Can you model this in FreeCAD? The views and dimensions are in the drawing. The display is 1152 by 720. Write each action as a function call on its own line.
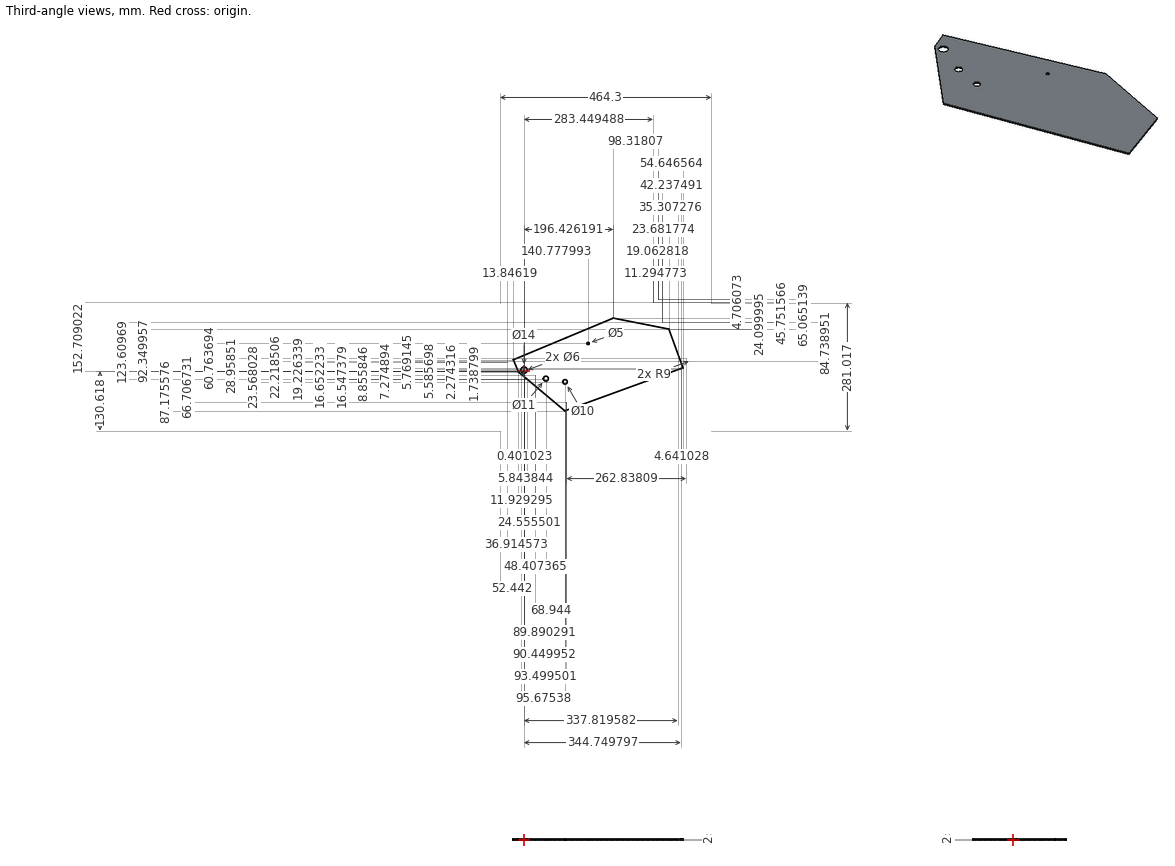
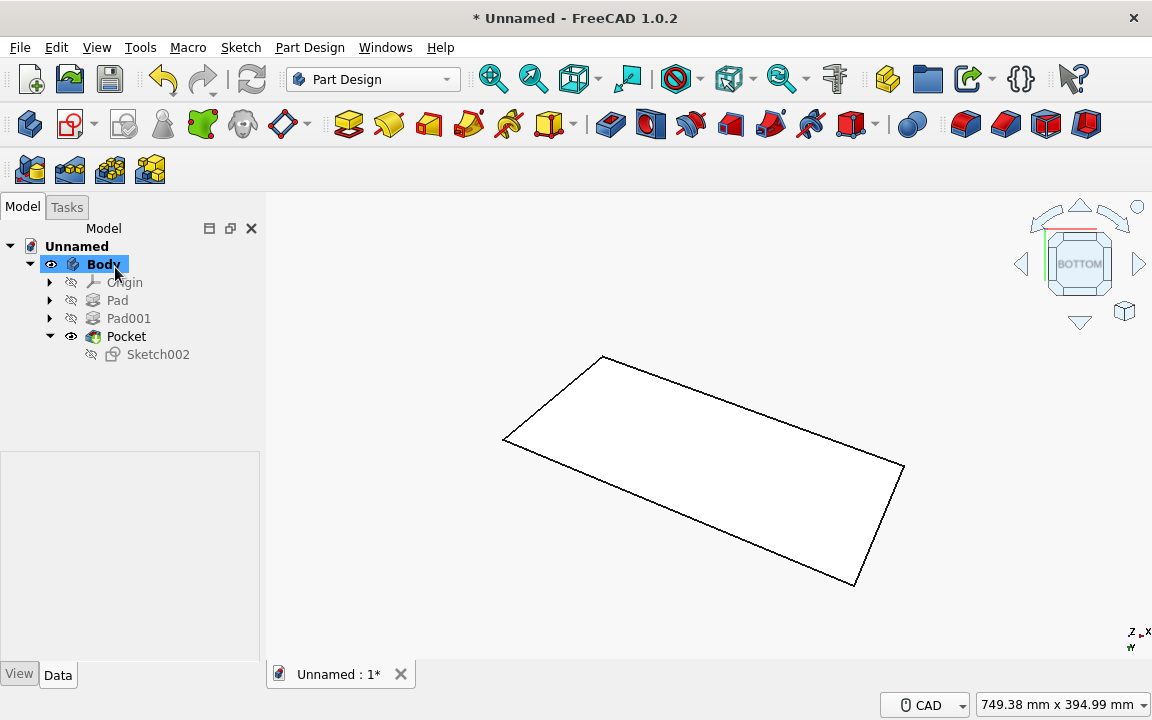
click(70, 124)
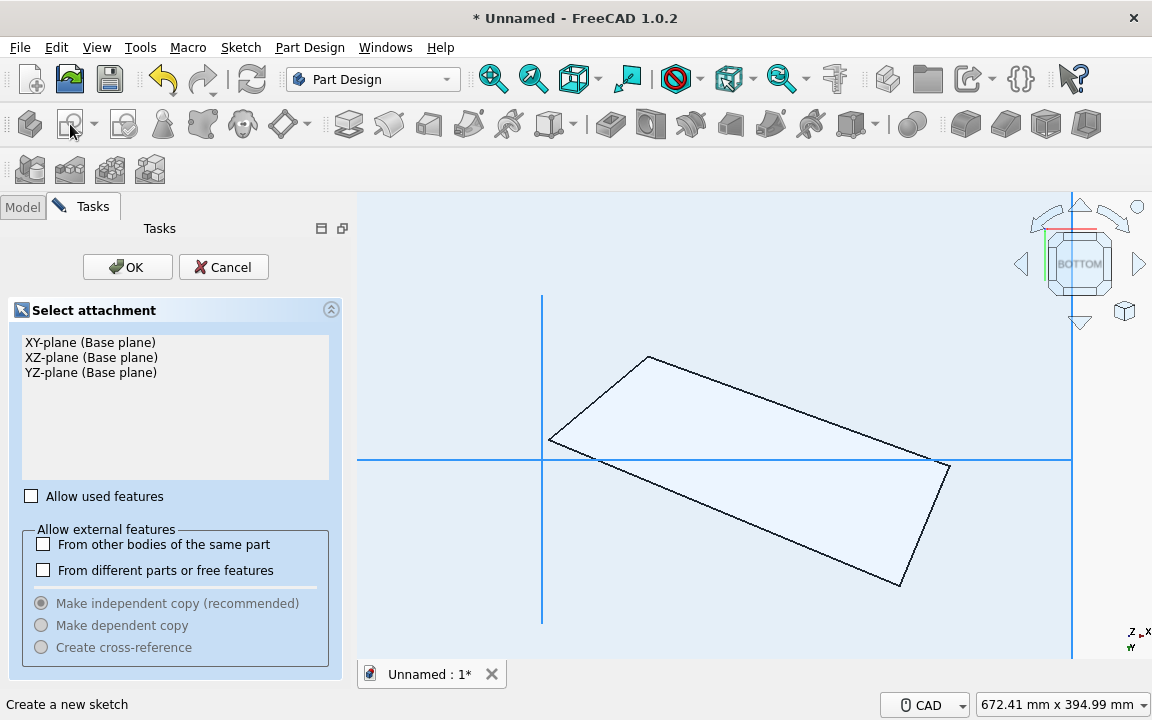
click(82, 342)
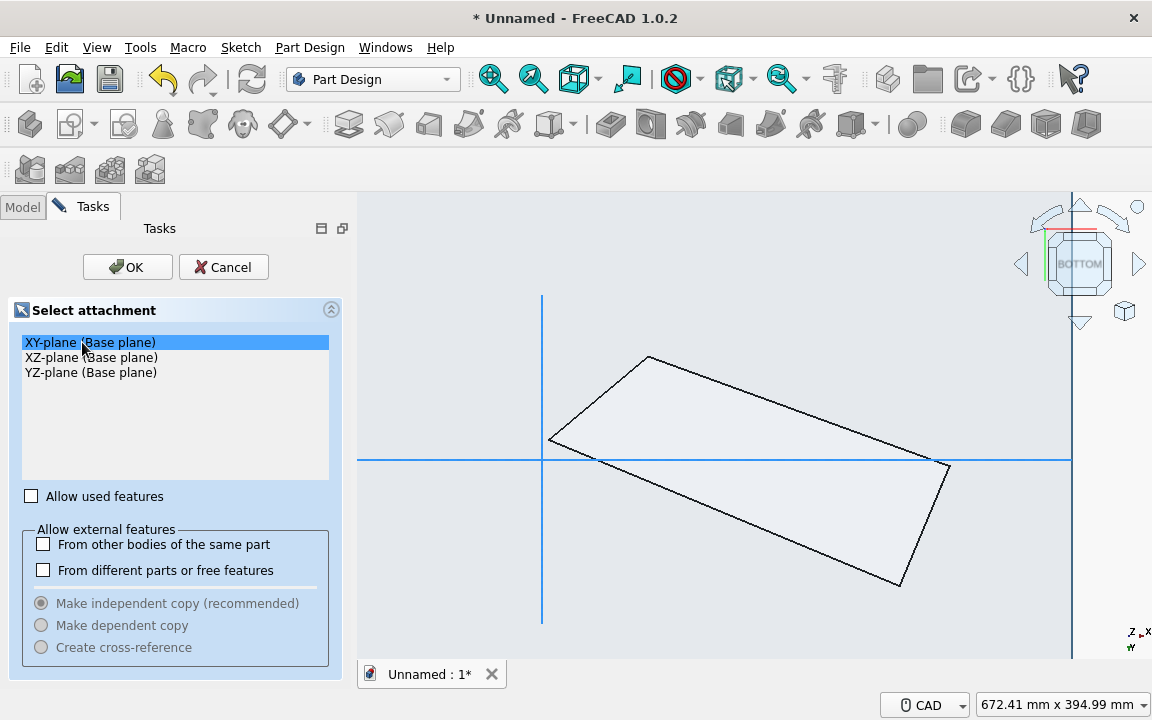
click(128, 267)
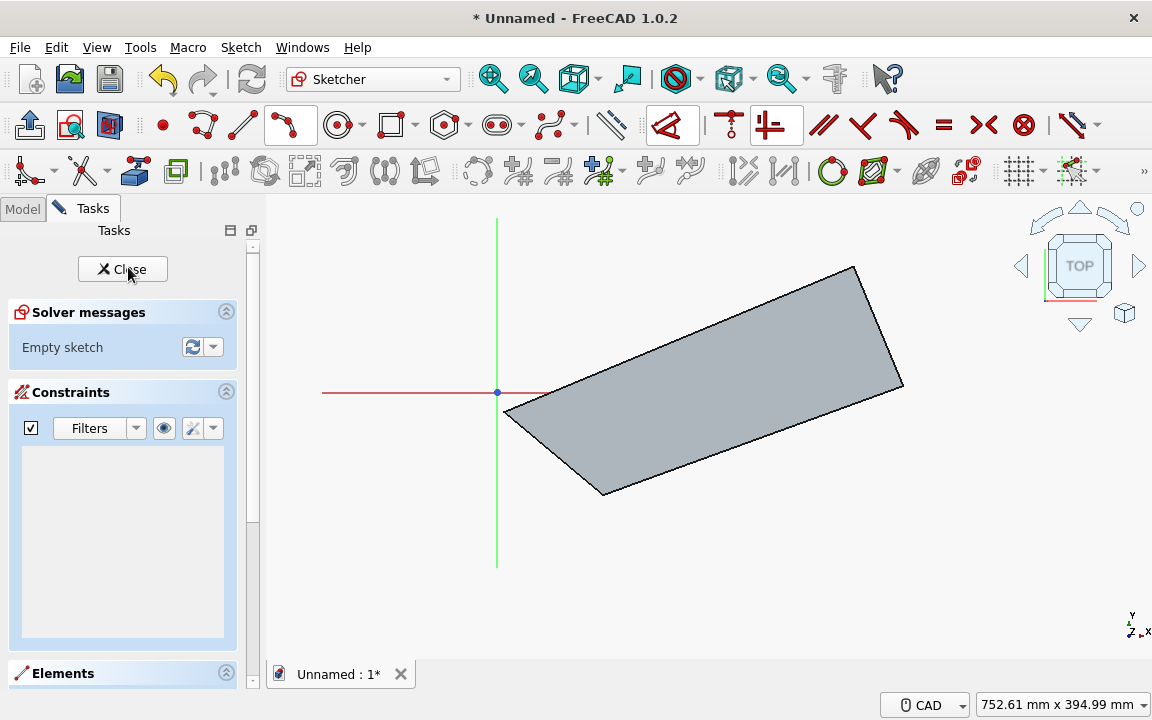
key(q)
key(s)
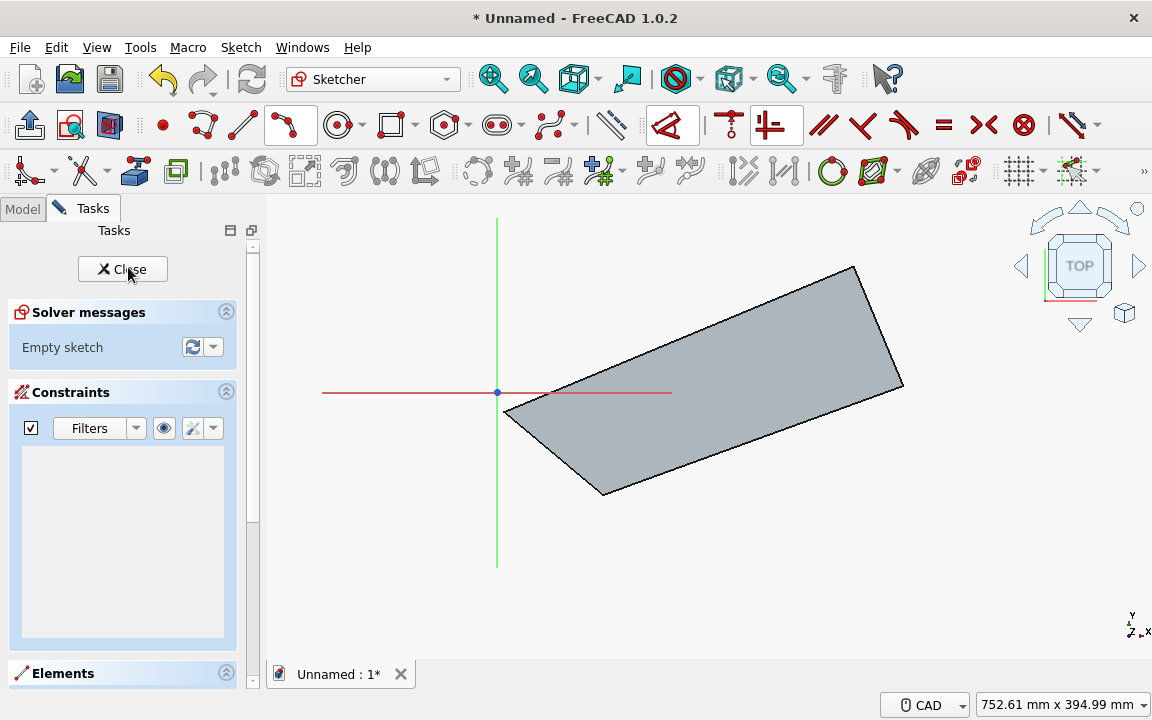
scroll(581, 631, down, 1)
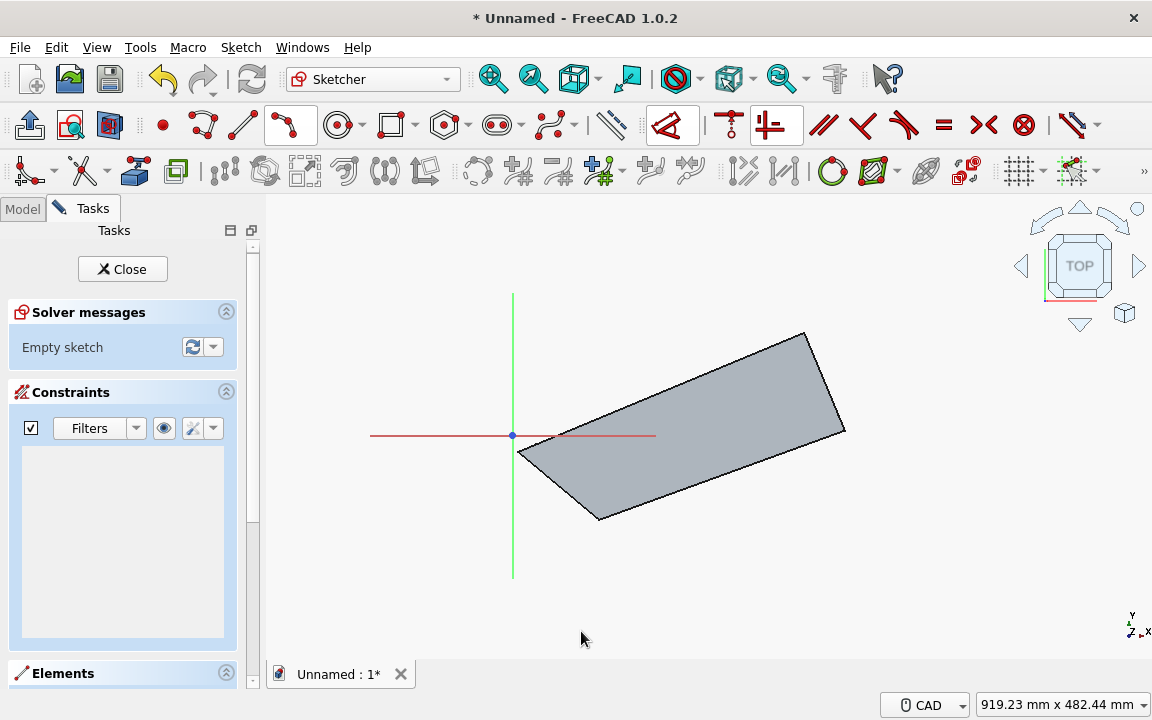
scroll(641, 256, up, 2)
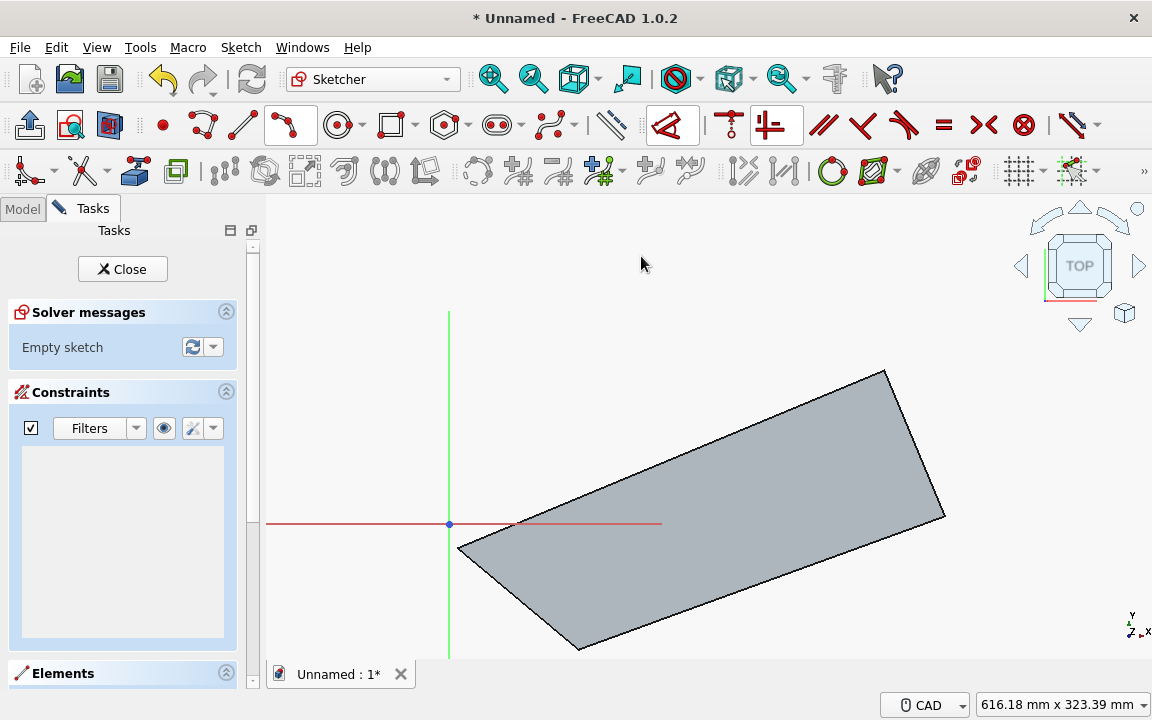
key(g)
key(m)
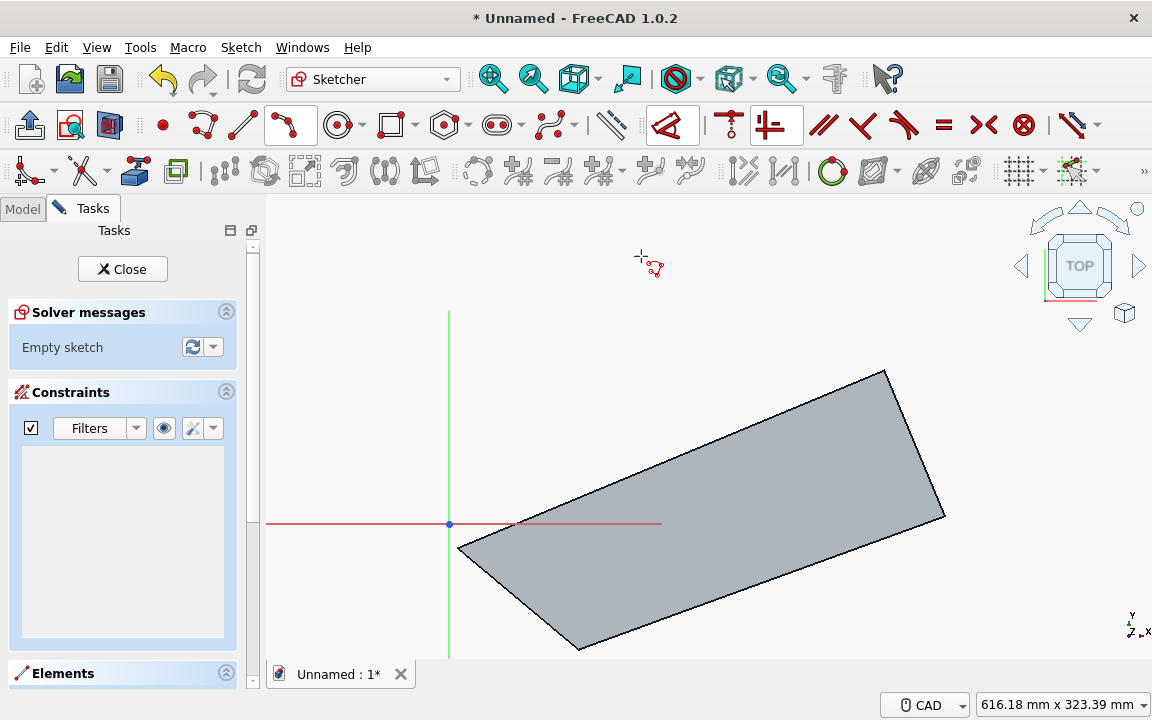
scroll(458, 548, up, 4)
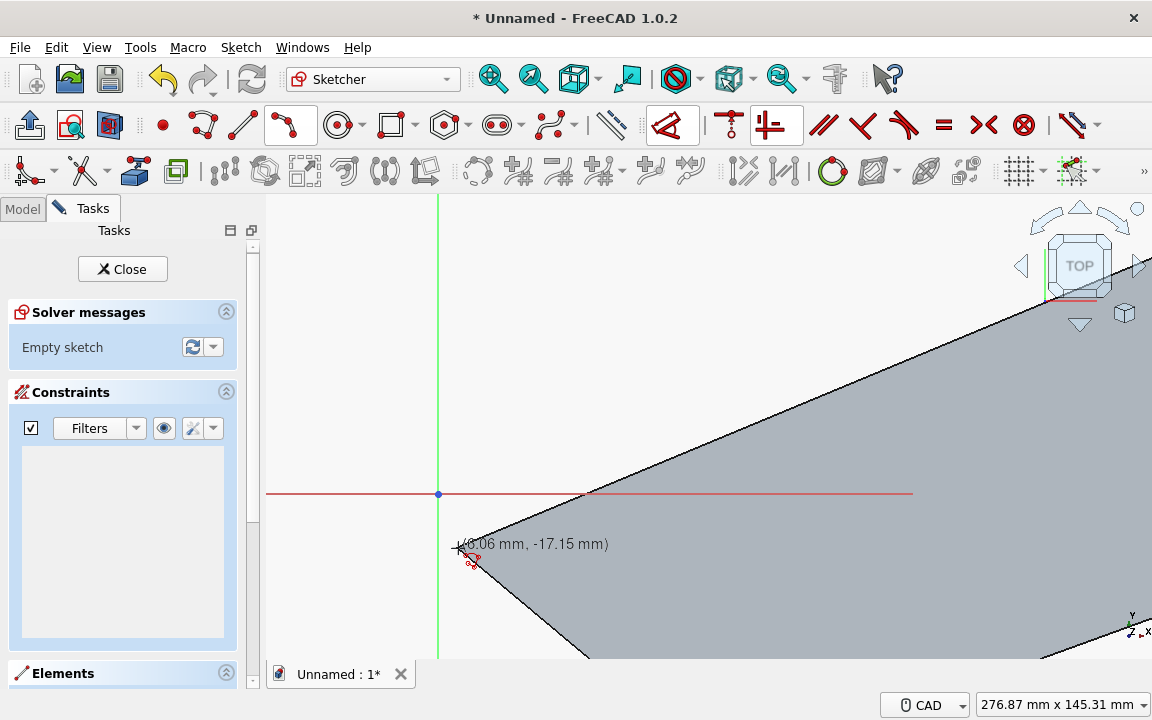
click(457, 548)
click(320, 433)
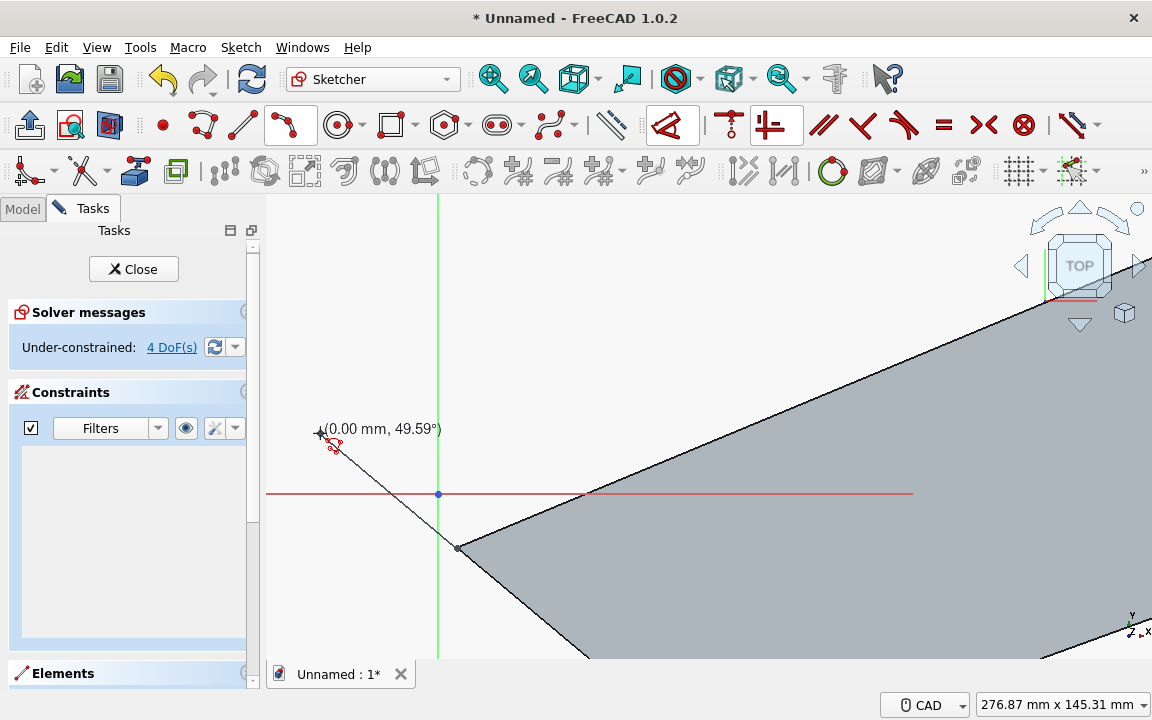
scroll(459, 549, down, 4)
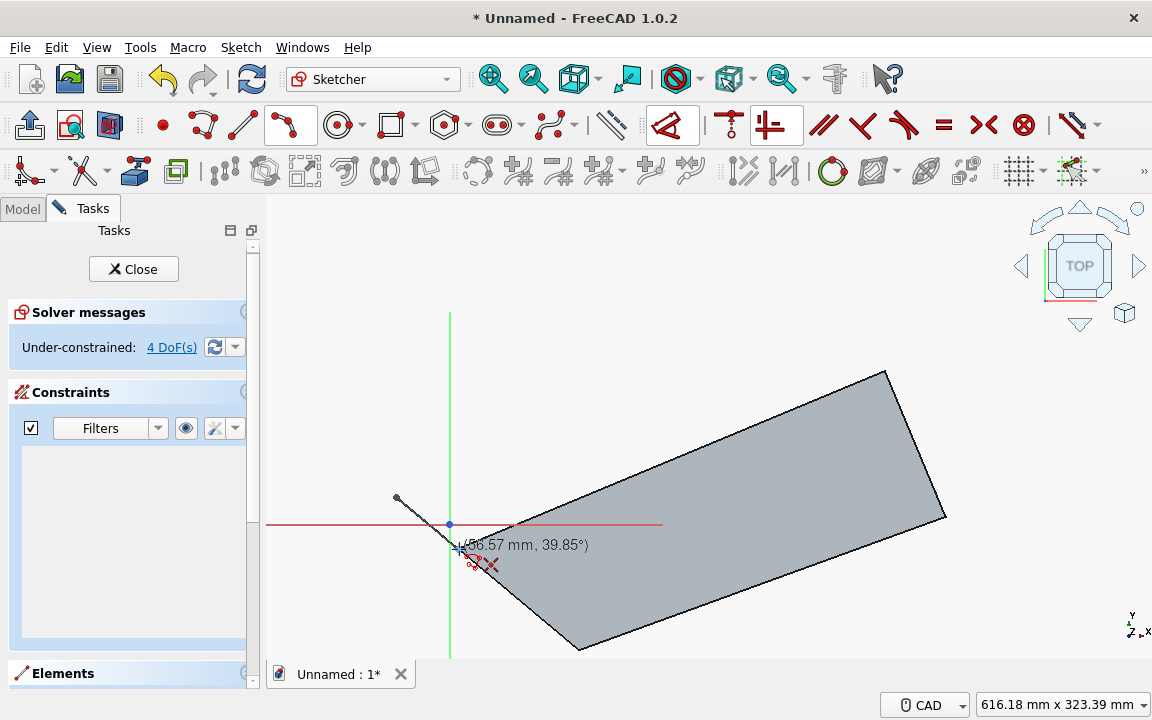
click(857, 305)
click(885, 371)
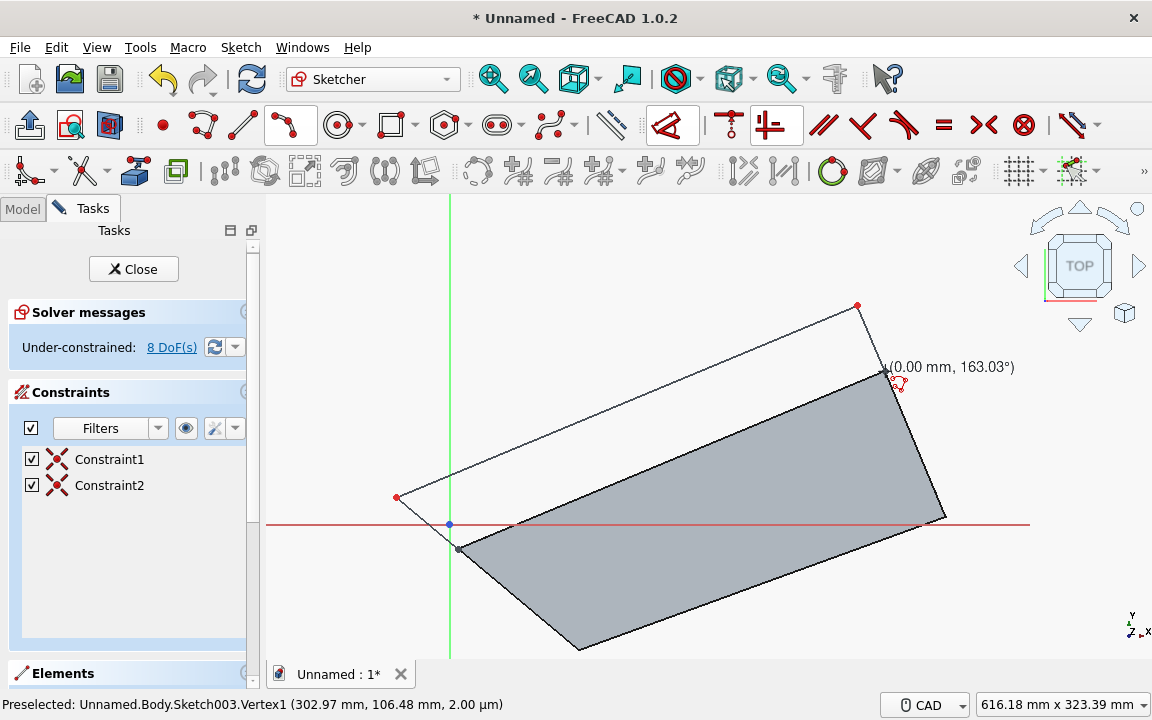
scroll(458, 549, up, 4)